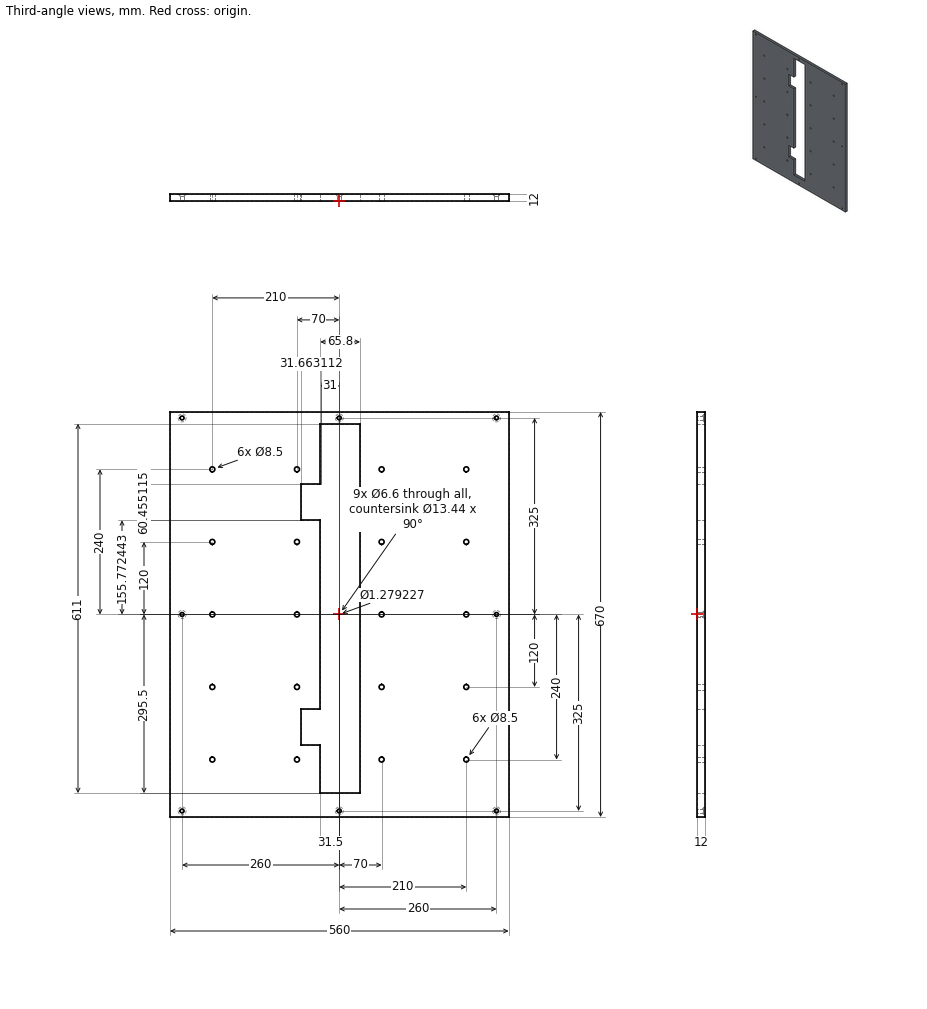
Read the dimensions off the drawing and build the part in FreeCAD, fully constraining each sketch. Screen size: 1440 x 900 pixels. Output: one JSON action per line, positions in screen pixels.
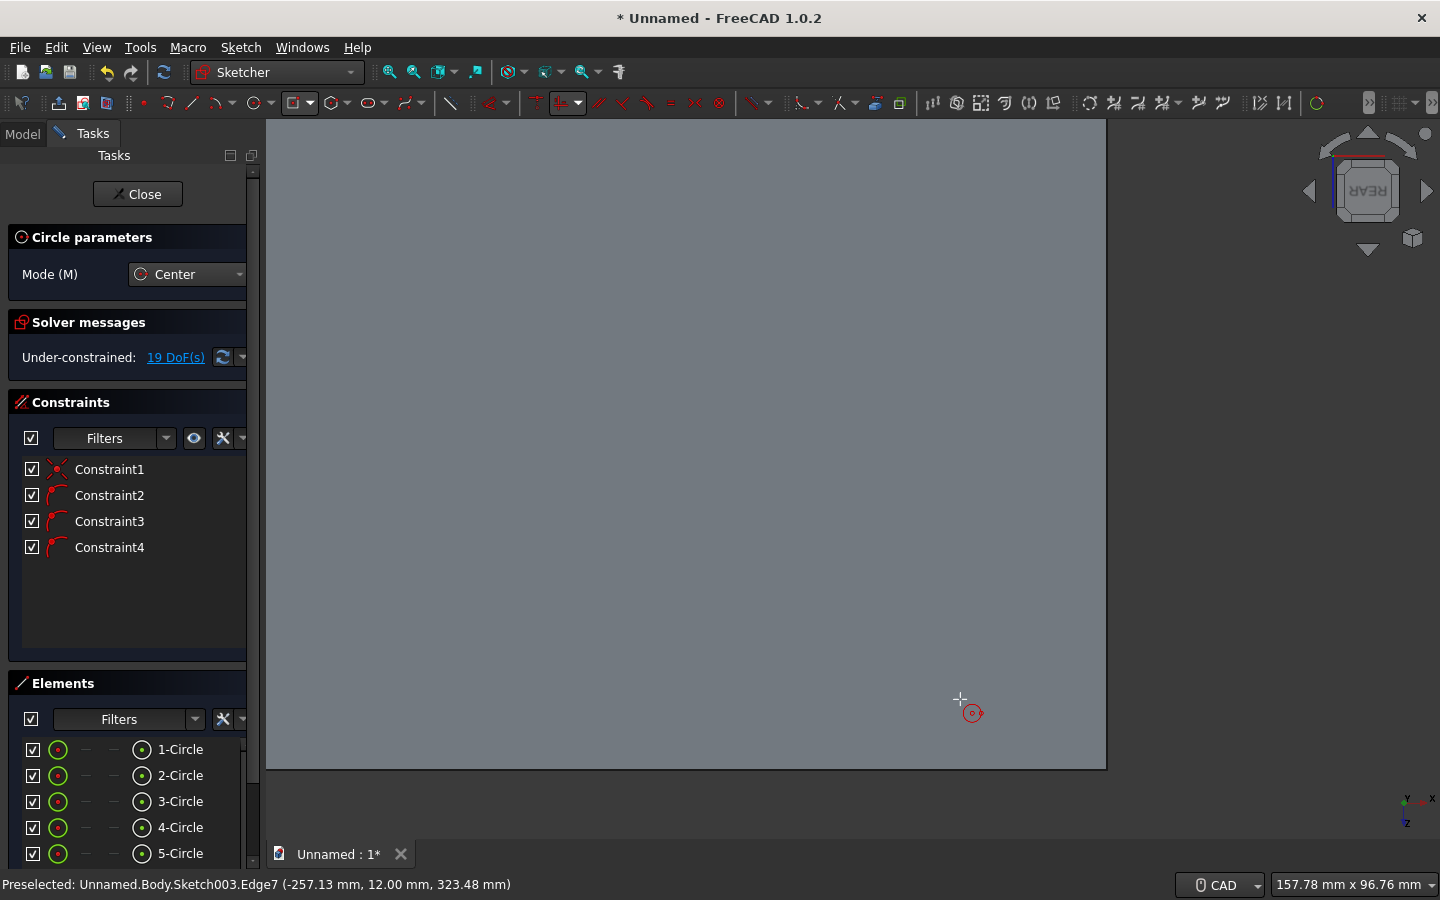
{"action": "scroll", "coordinate": [960, 699], "scroll_direction": "down", "scroll_amount": 12}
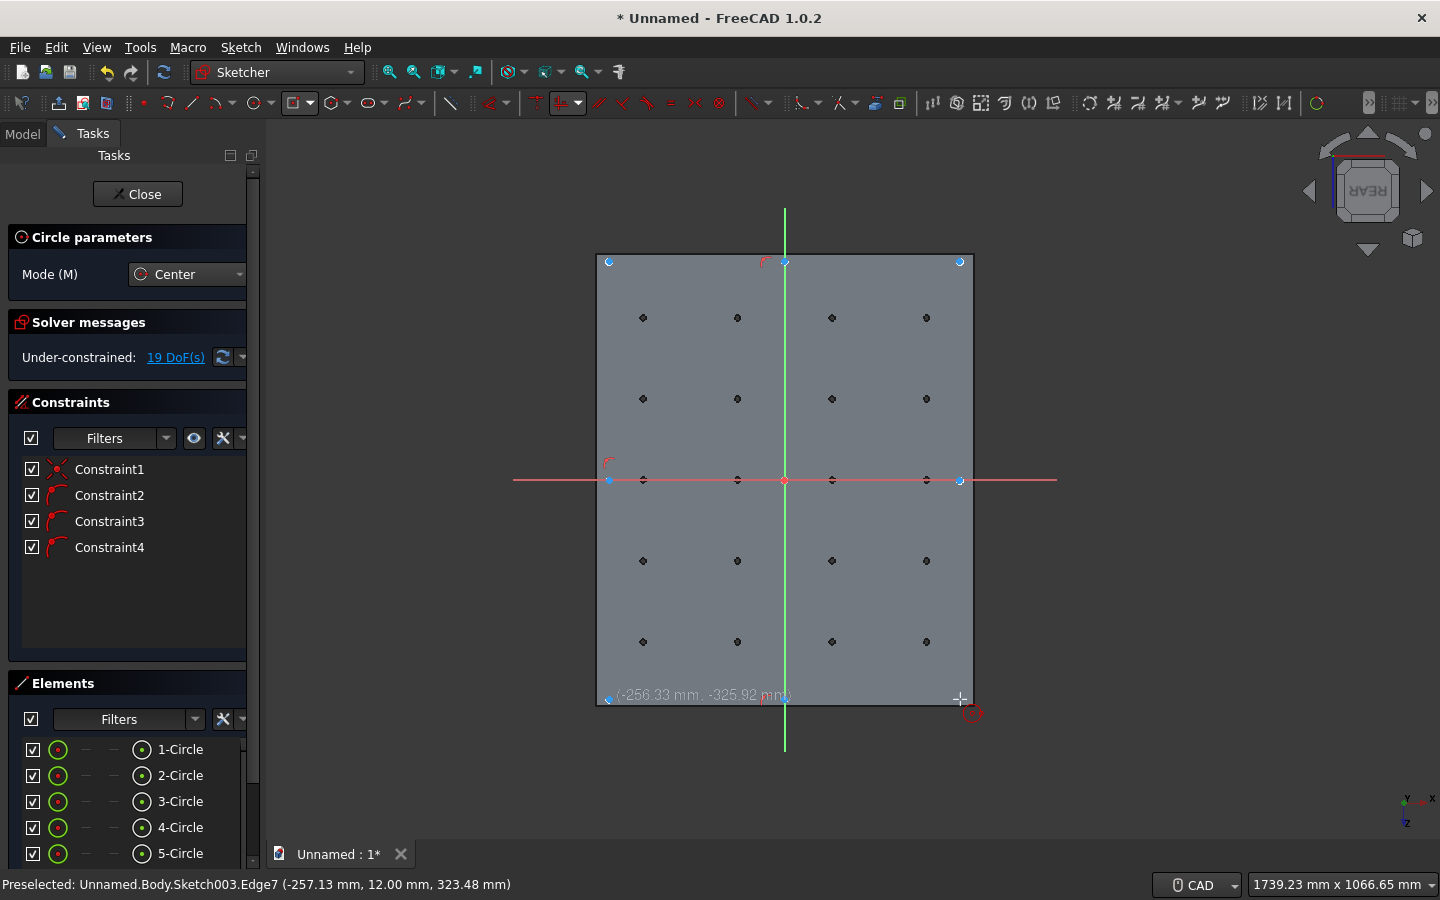
{"action": "left_click", "coordinate": [960, 699]}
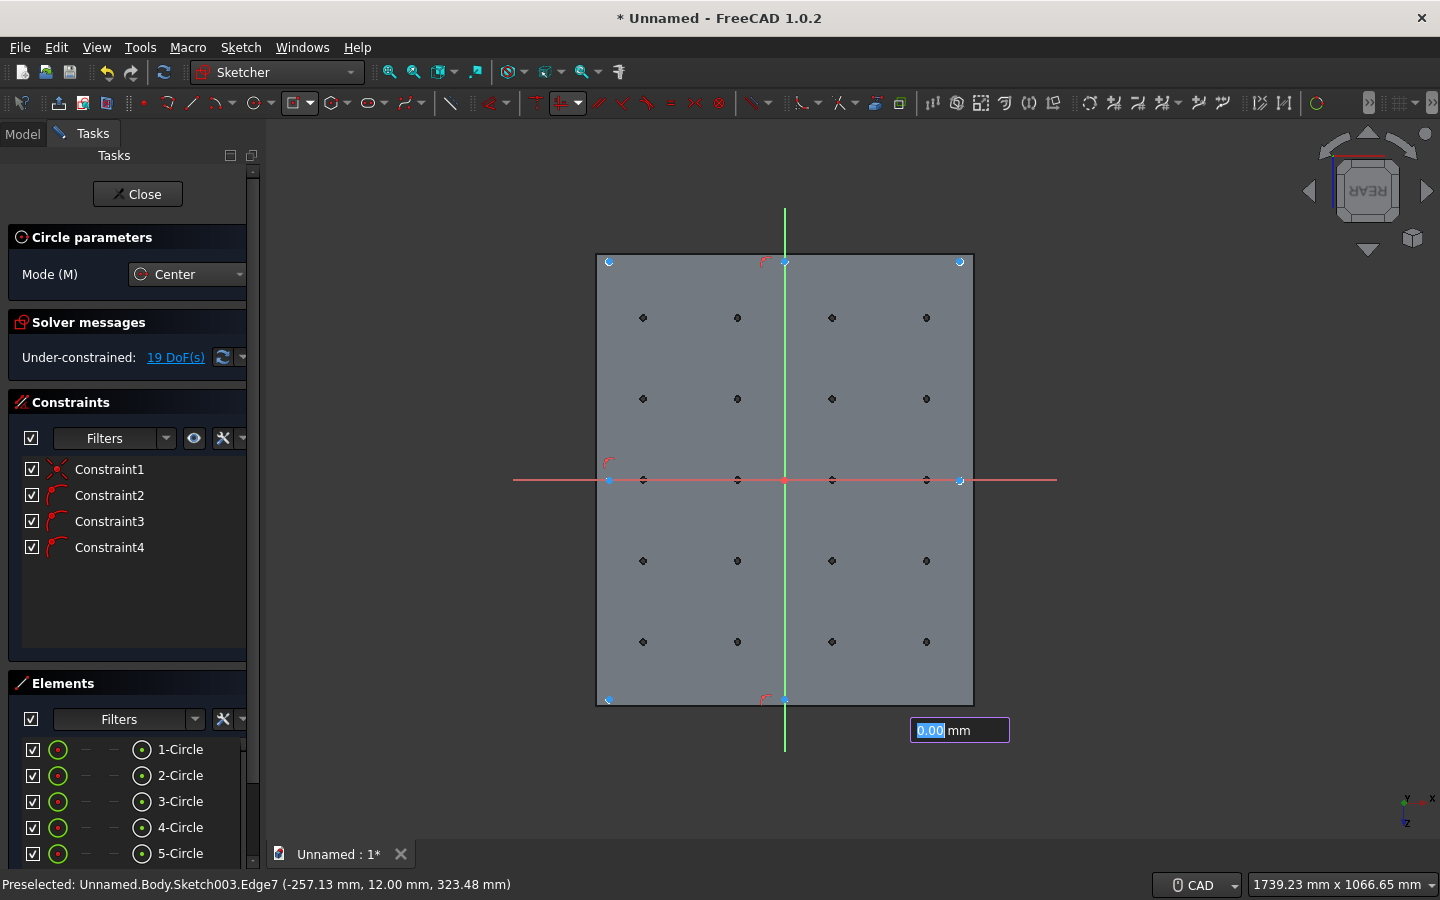
{"action": "scroll", "coordinate": [962, 698], "scroll_direction": "up", "scroll_amount": 10}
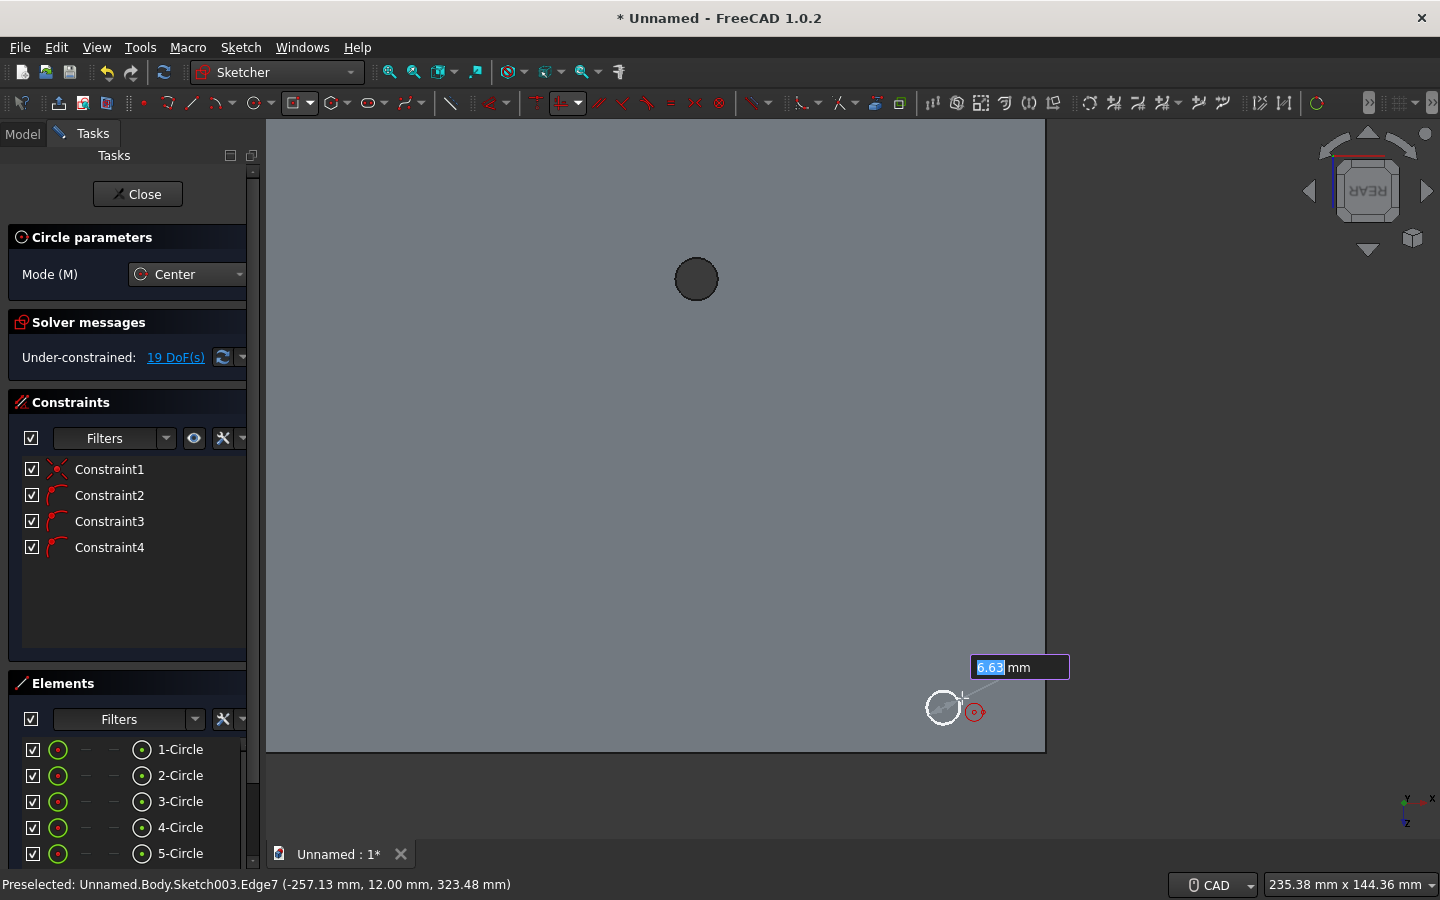
{"action": "left_click", "coordinate": [958, 691]}
{"action": "key", "text": "Escape"}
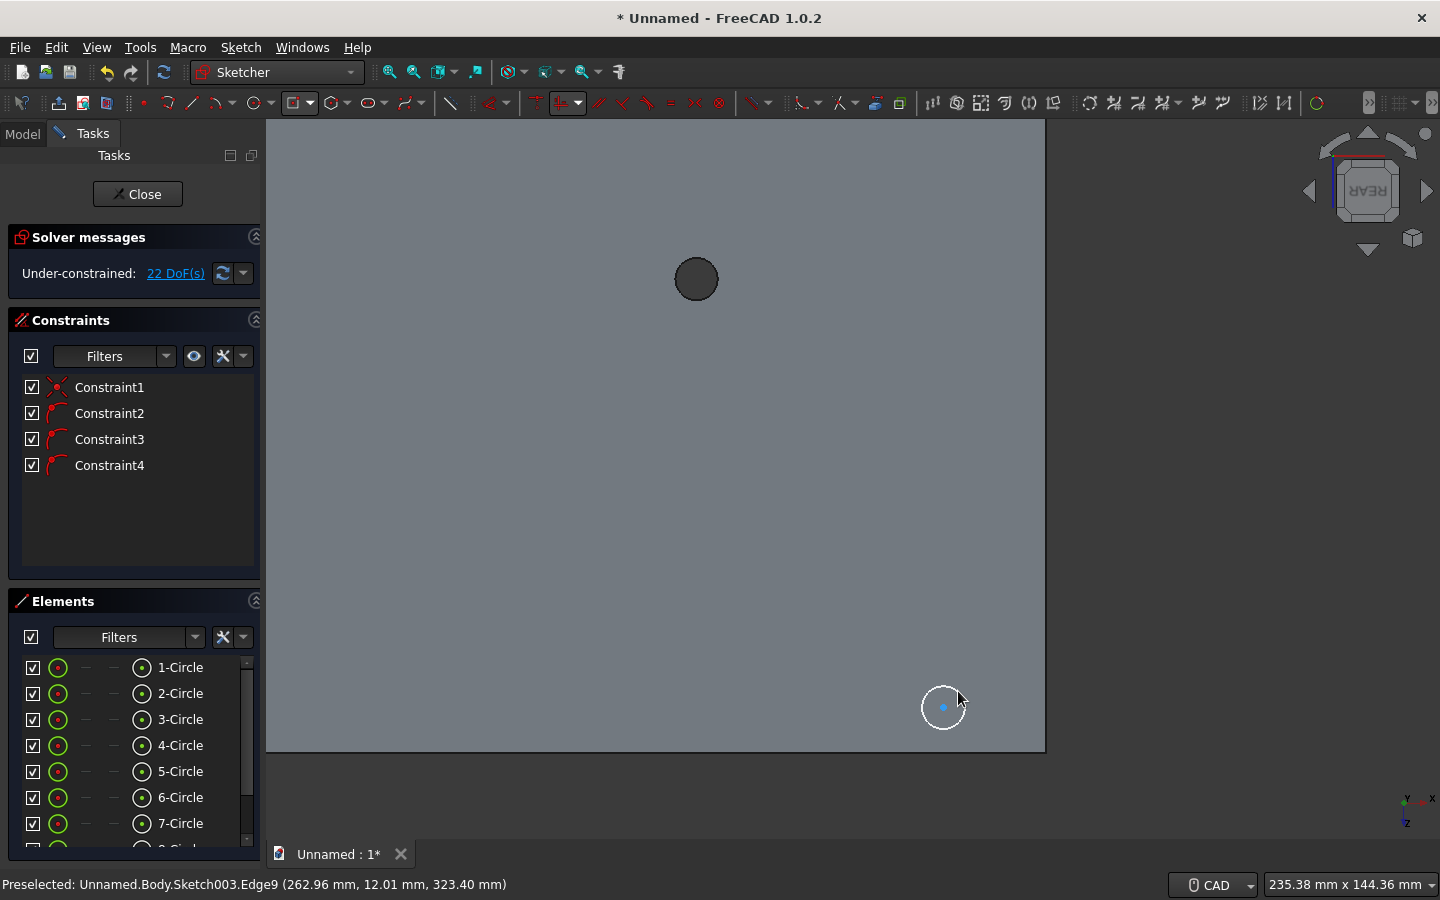
{"action": "scroll", "coordinate": [962, 698], "scroll_direction": "down", "scroll_amount": 10}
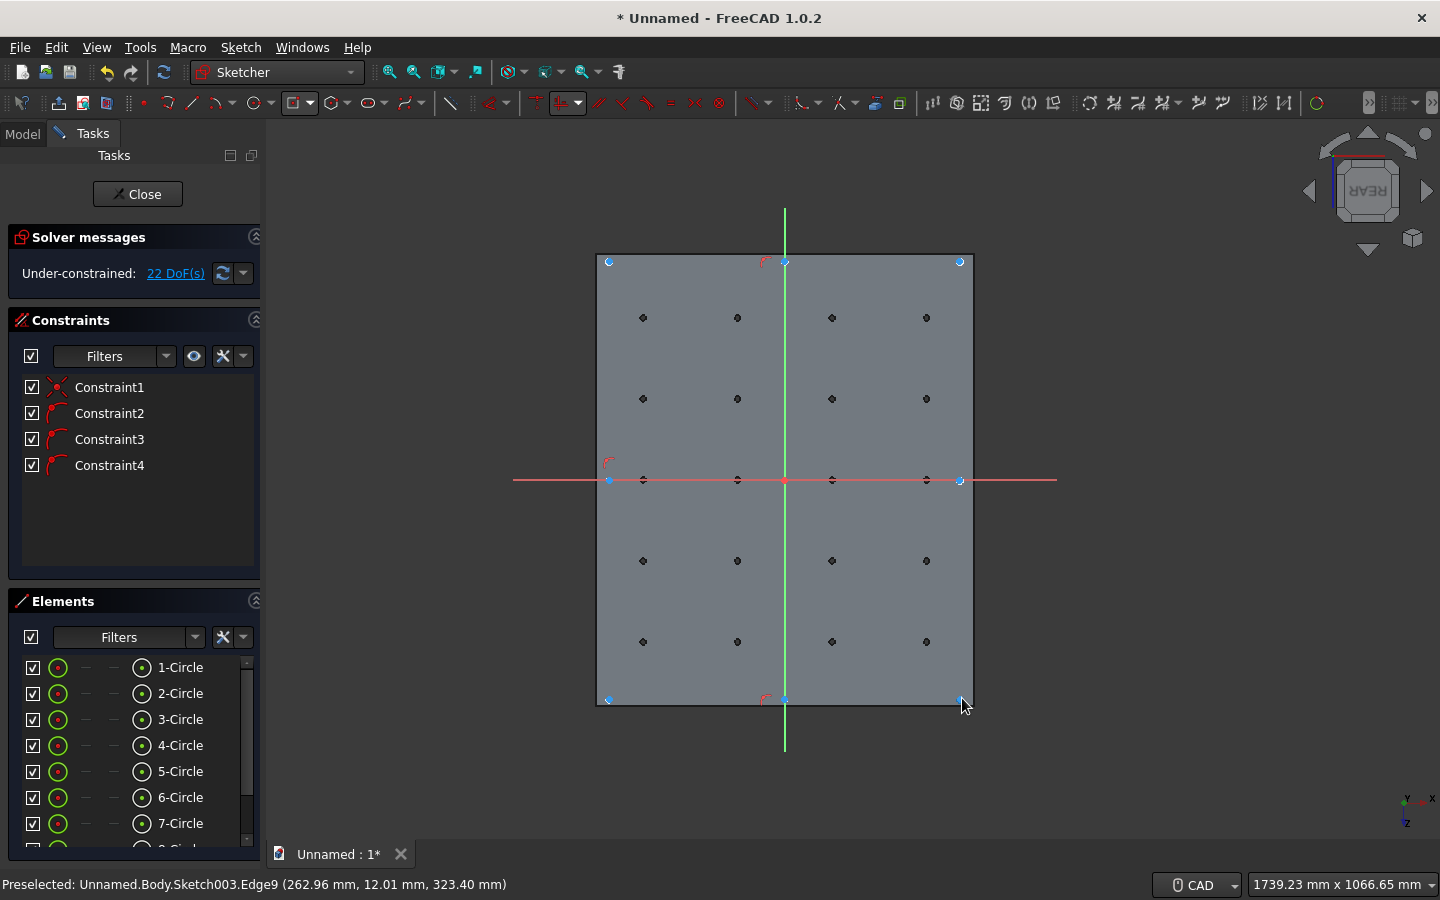
{"action": "scroll", "coordinate": [786, 478], "scroll_direction": "up", "scroll_amount": 12}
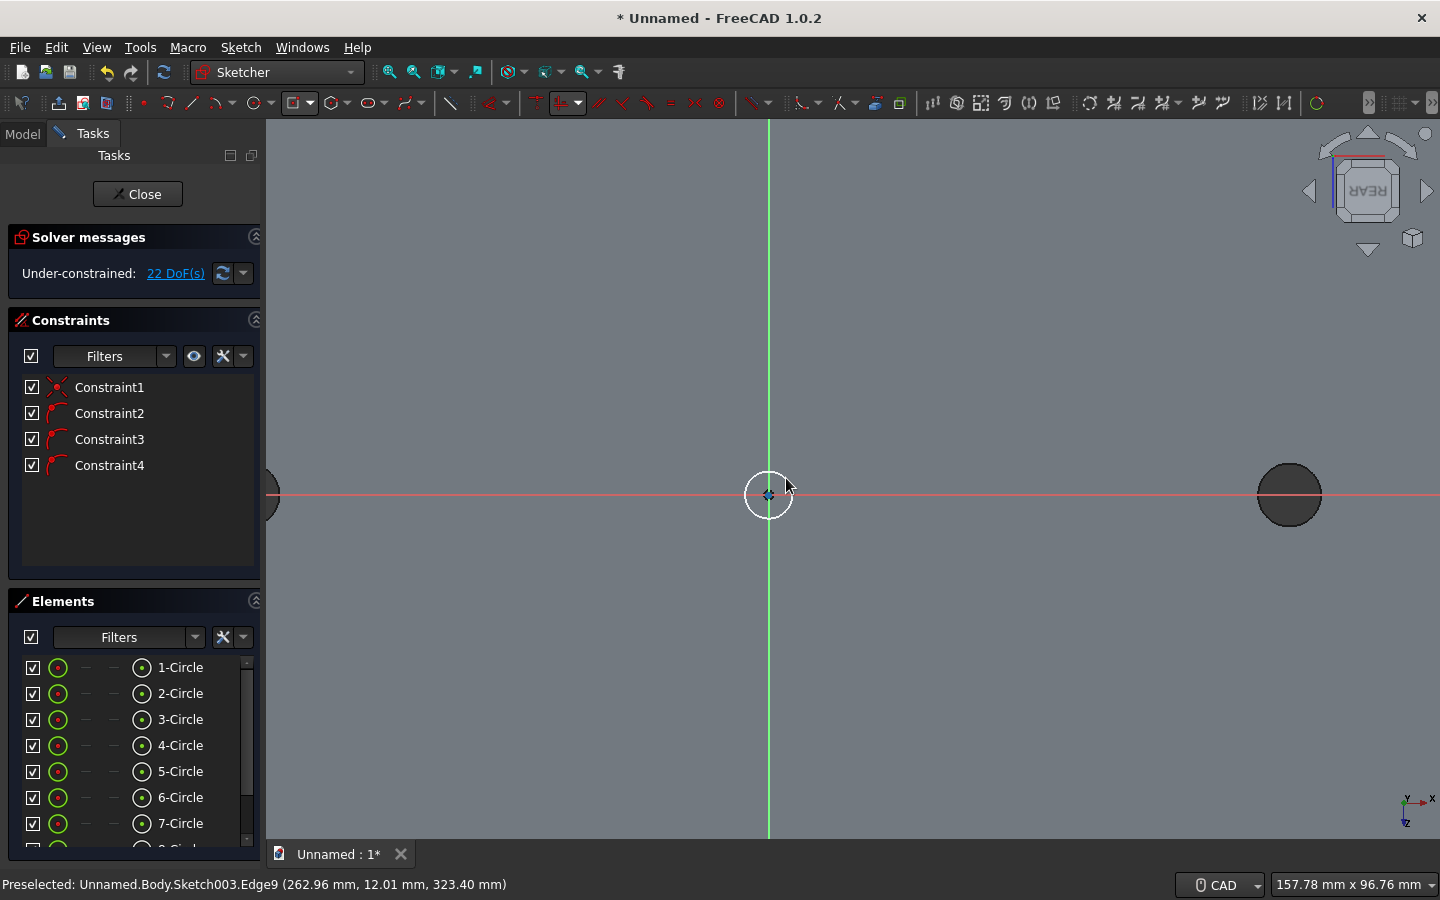
{"action": "left_click", "coordinate": [785, 478]}